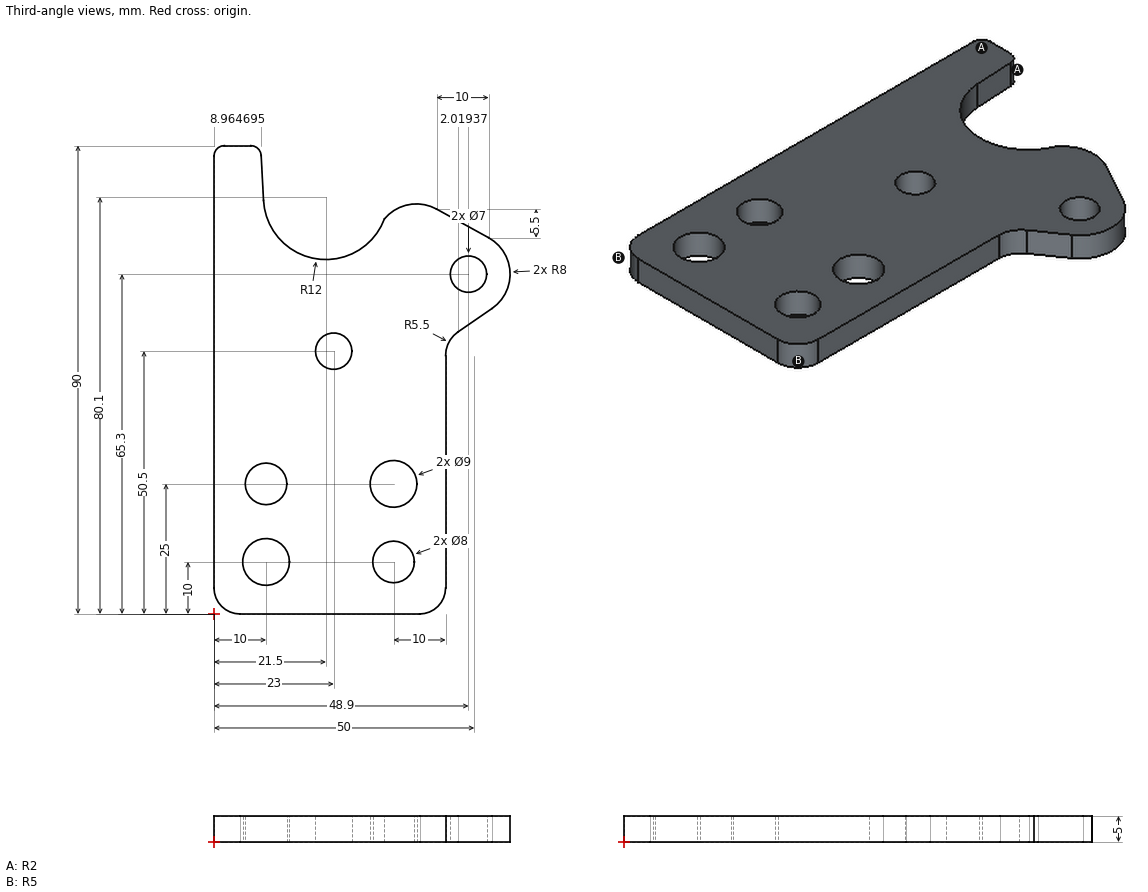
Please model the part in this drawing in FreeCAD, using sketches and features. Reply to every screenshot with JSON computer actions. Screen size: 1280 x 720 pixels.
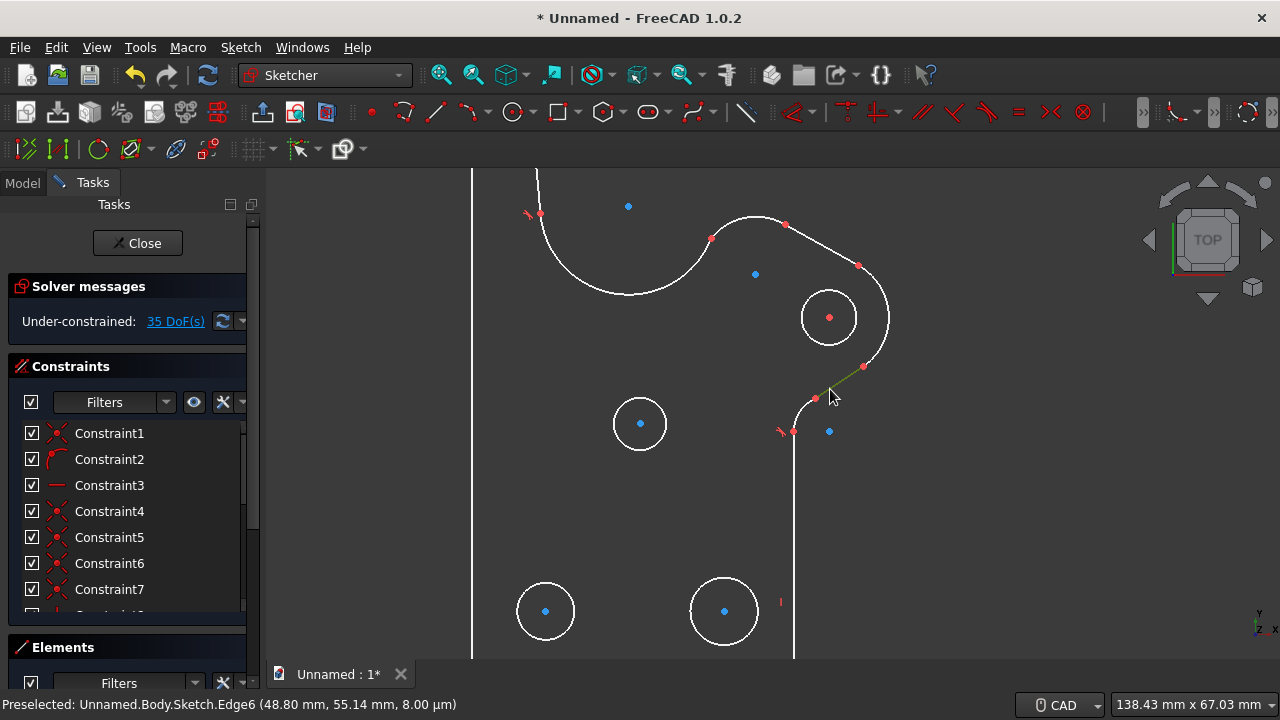
{"action": "left_click", "coordinate": [805, 406]}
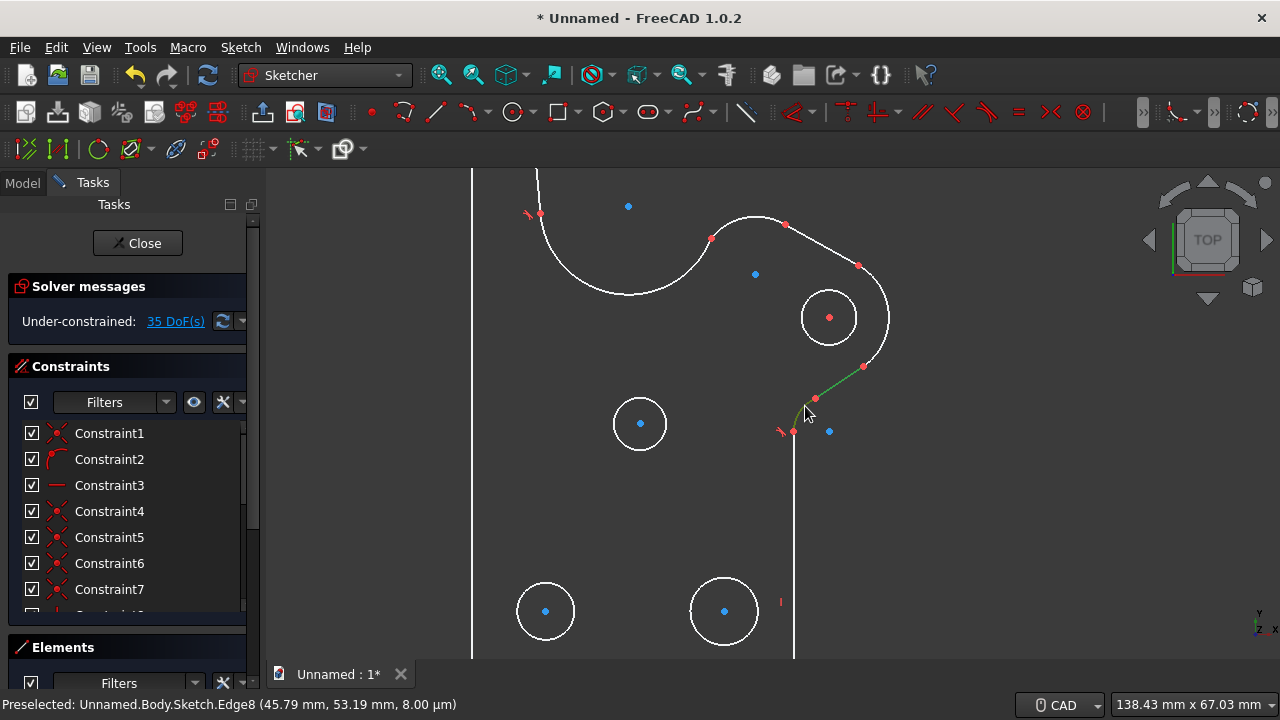
{"action": "key", "text": "t"}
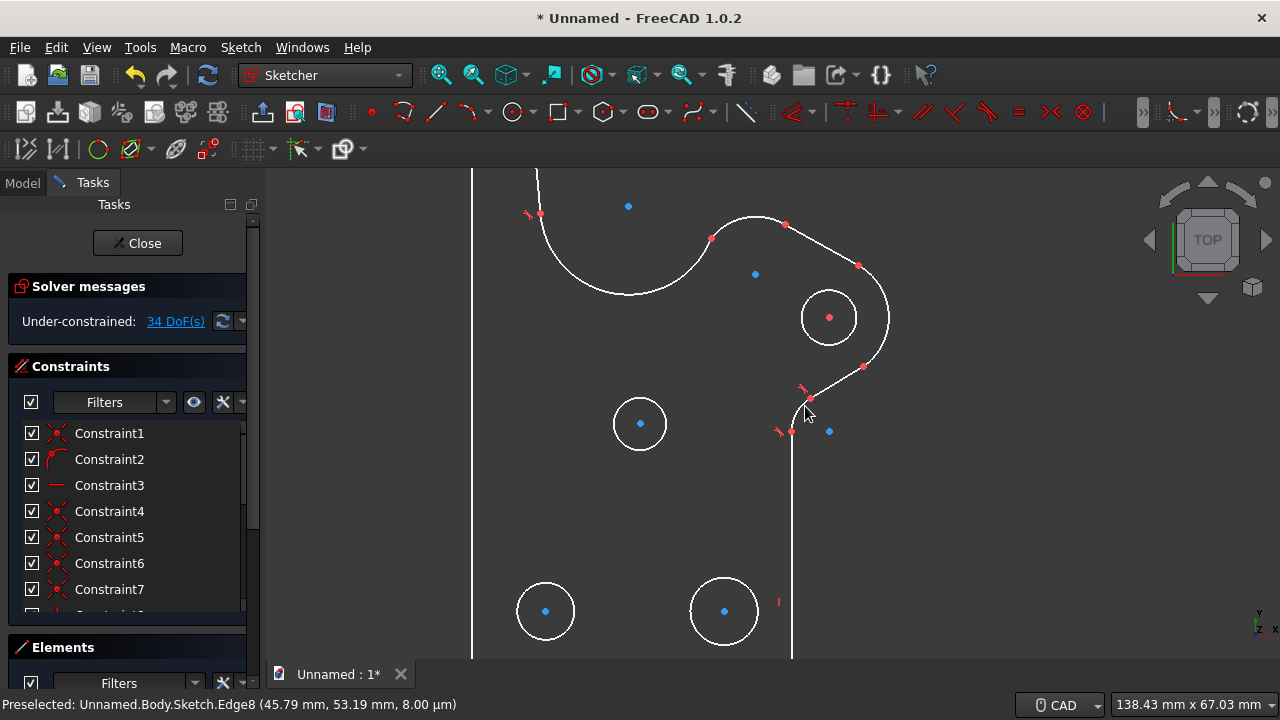
{"action": "left_click", "coordinate": [826, 389]}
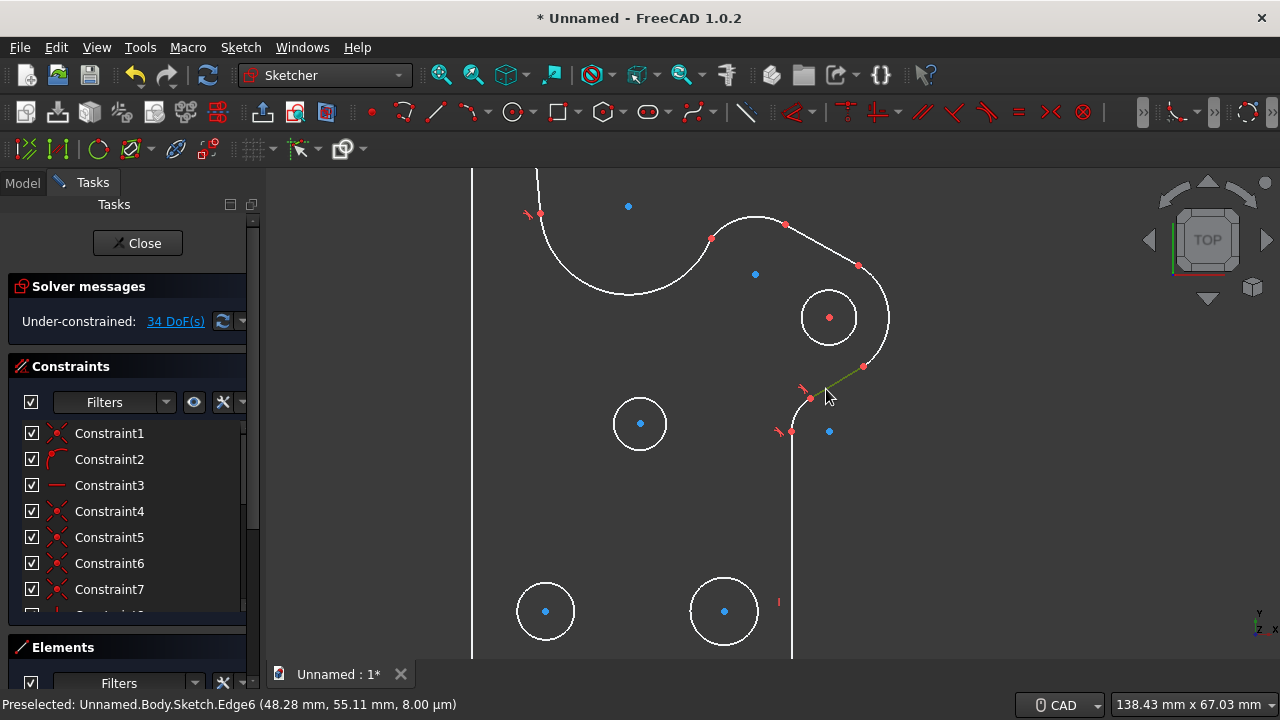
{"action": "left_click", "coordinate": [885, 338]}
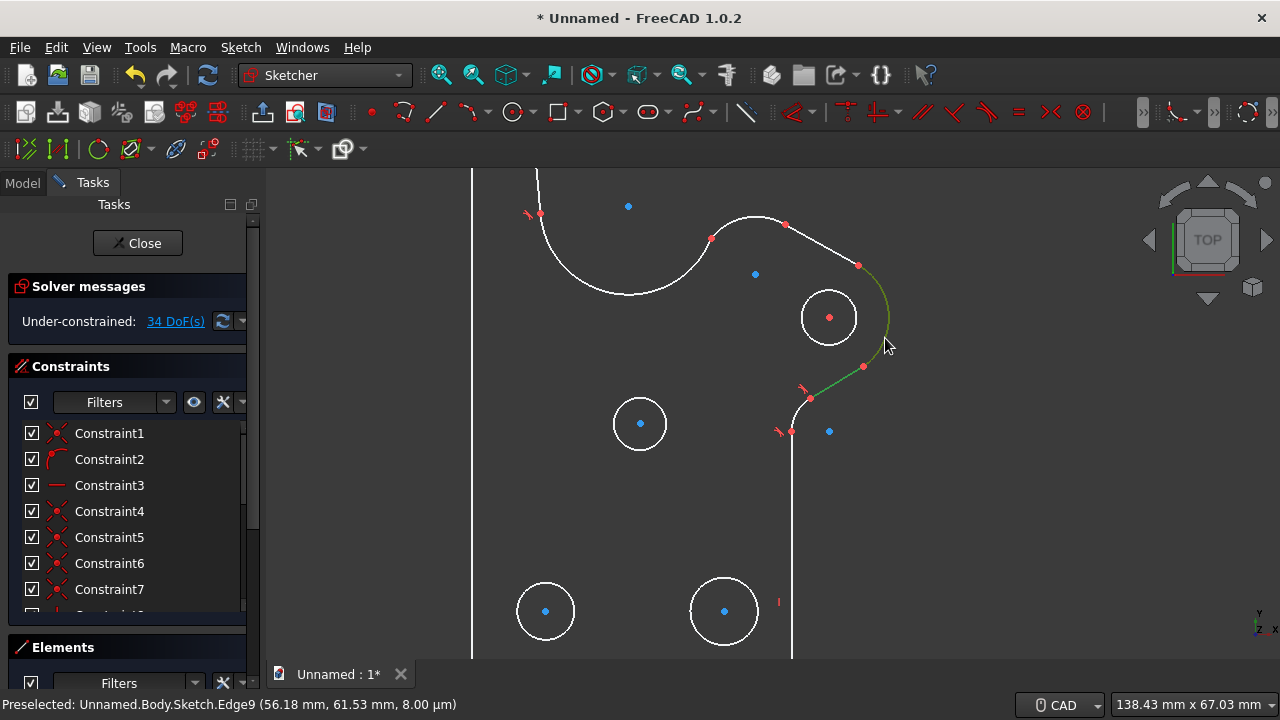
{"action": "key", "text": "t"}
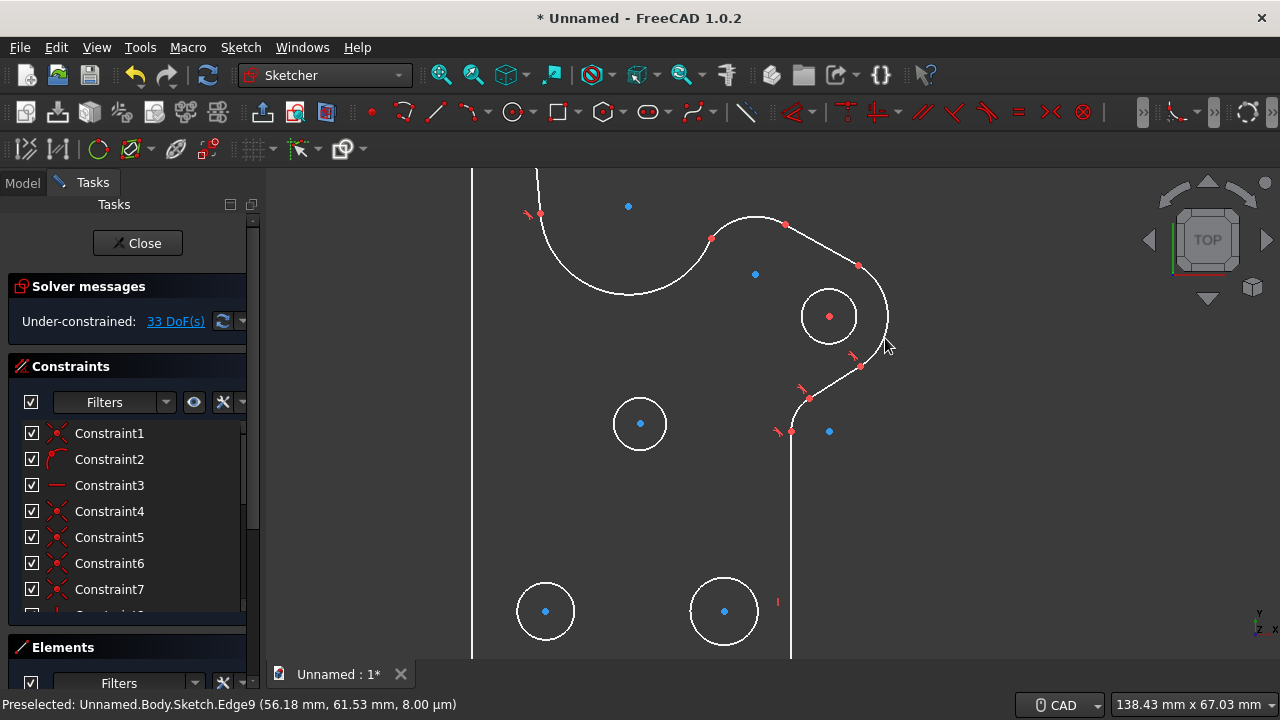
{"action": "left_click", "coordinate": [836, 253]}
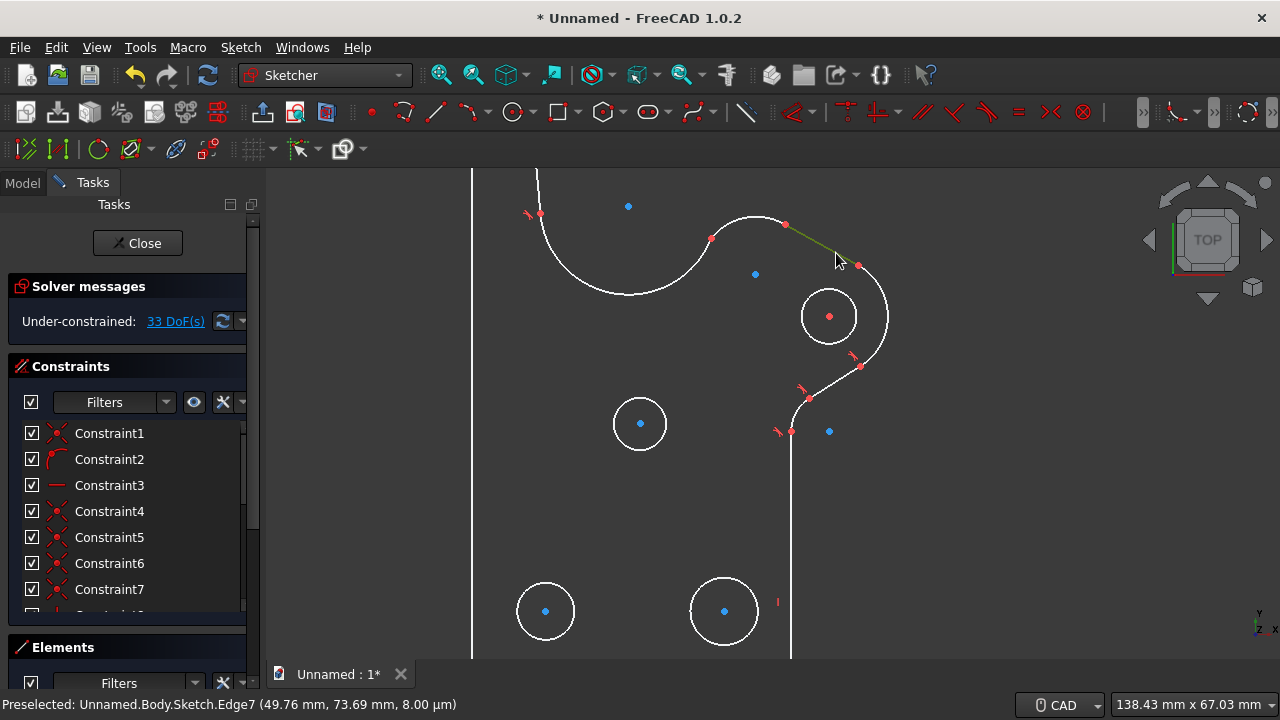
{"action": "left_click", "coordinate": [883, 339]}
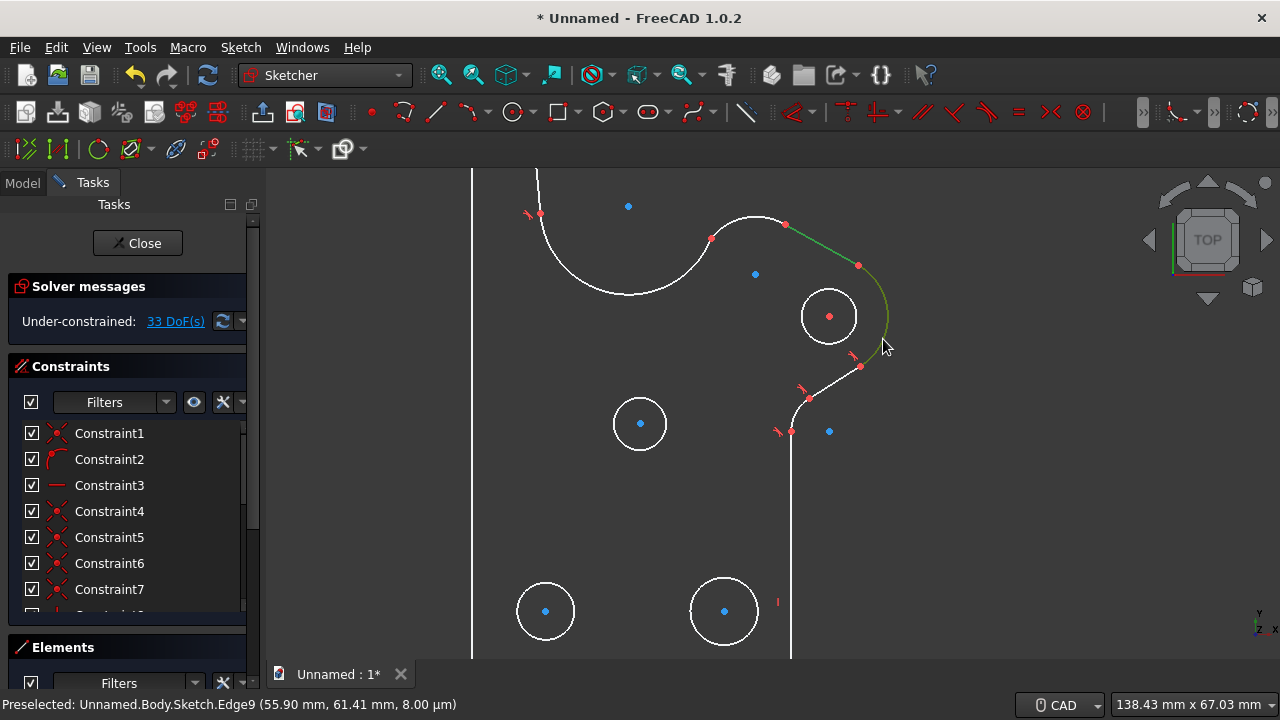
{"action": "key", "text": "t"}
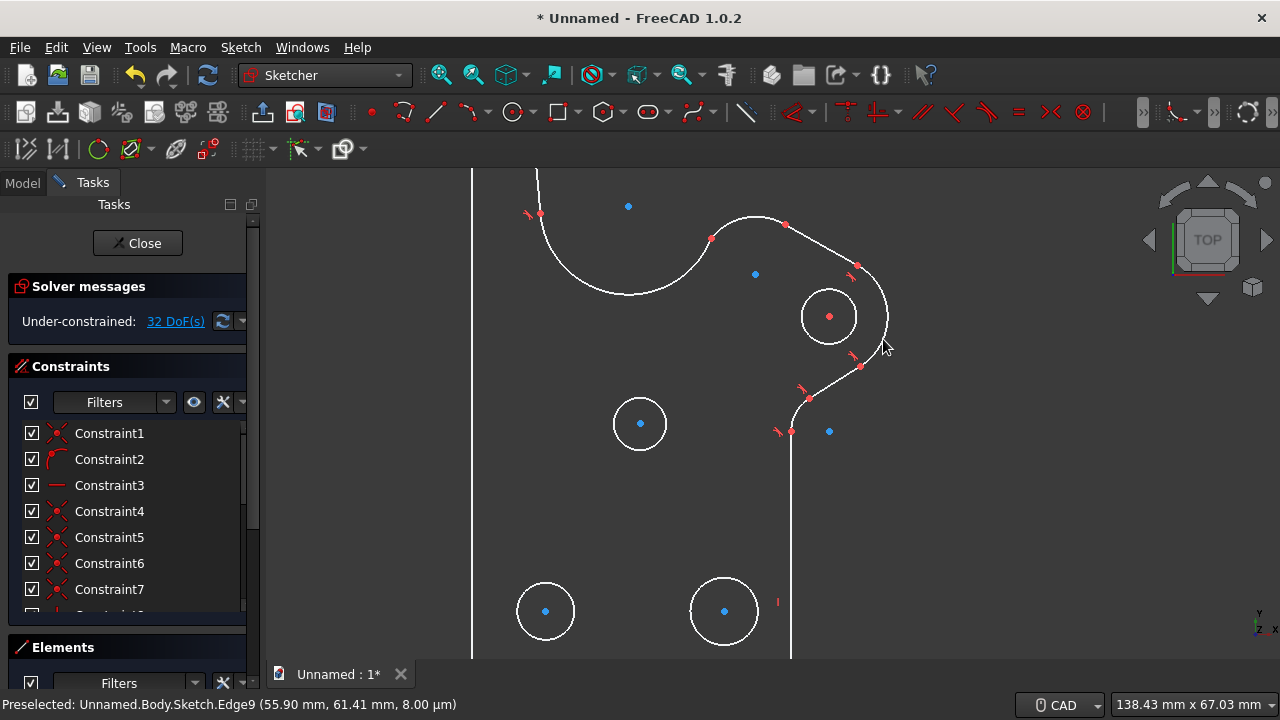
{"action": "left_click", "coordinate": [836, 253]}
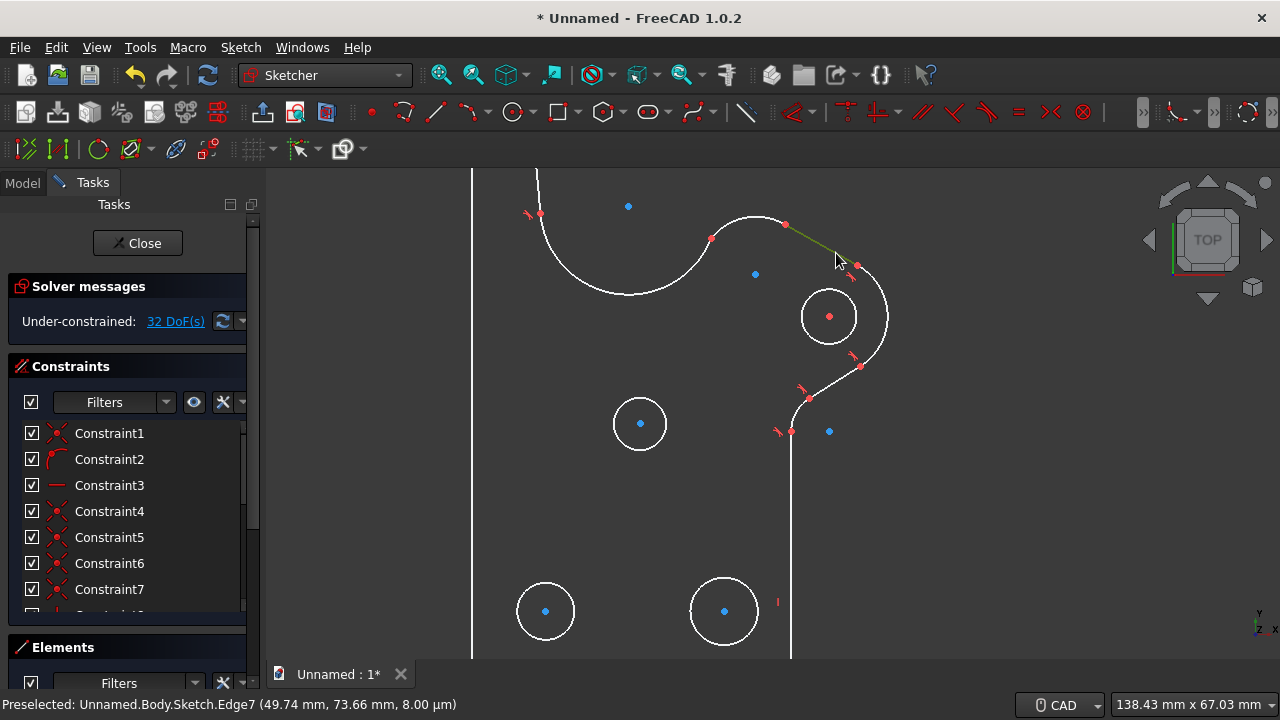
{"action": "left_click", "coordinate": [762, 217]}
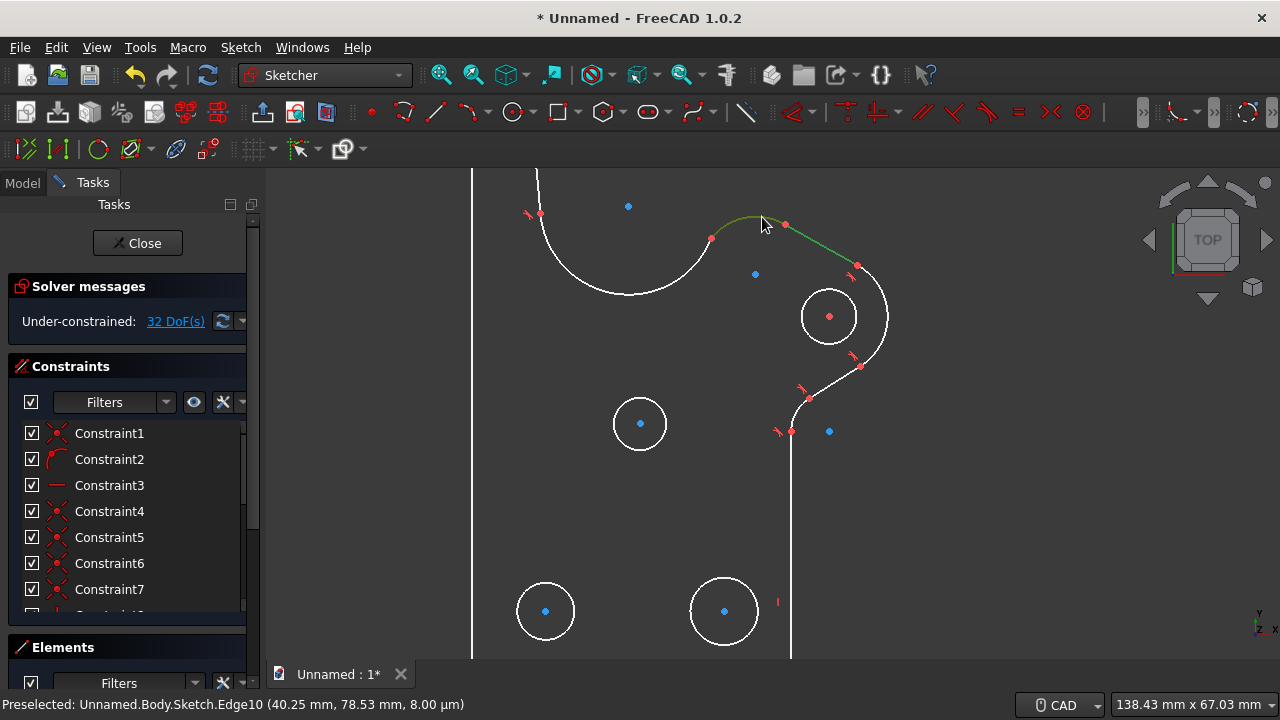
{"action": "key", "text": "t"}